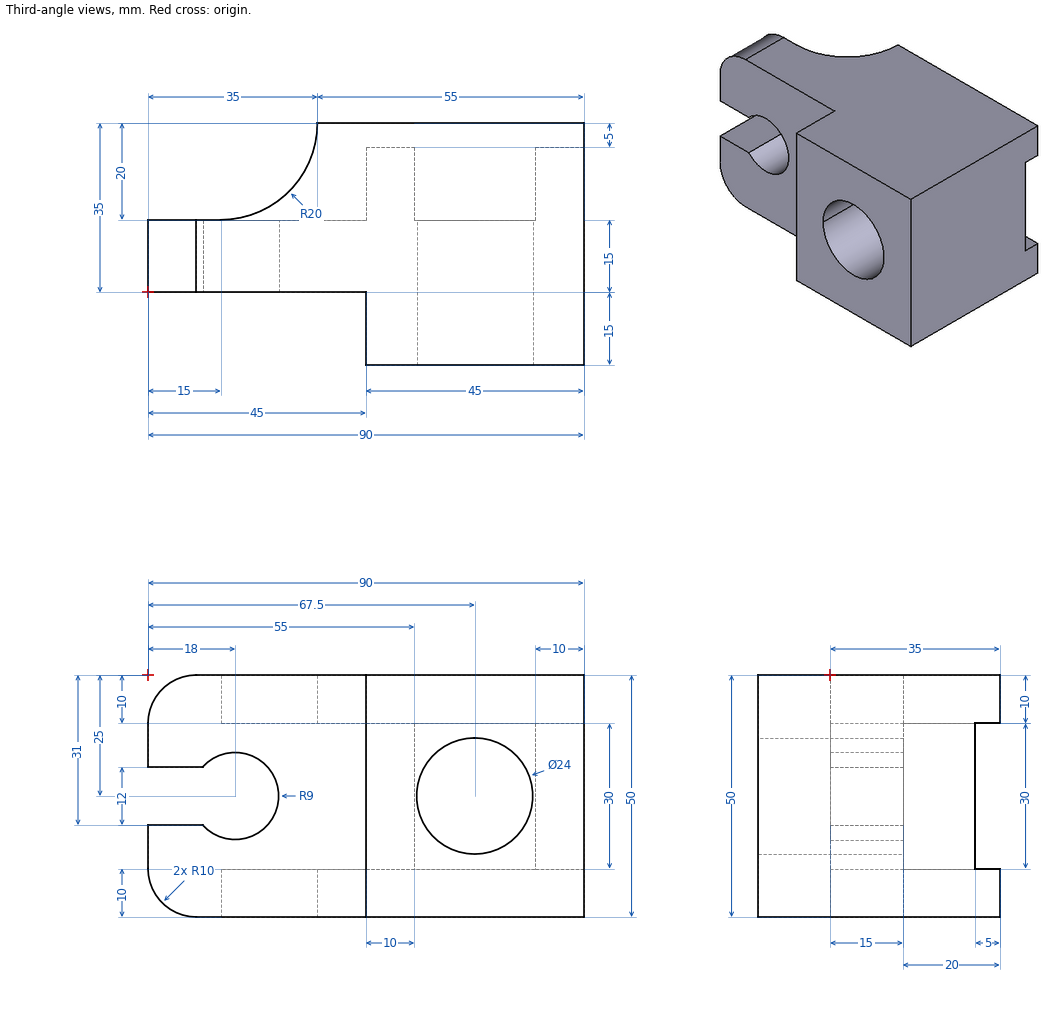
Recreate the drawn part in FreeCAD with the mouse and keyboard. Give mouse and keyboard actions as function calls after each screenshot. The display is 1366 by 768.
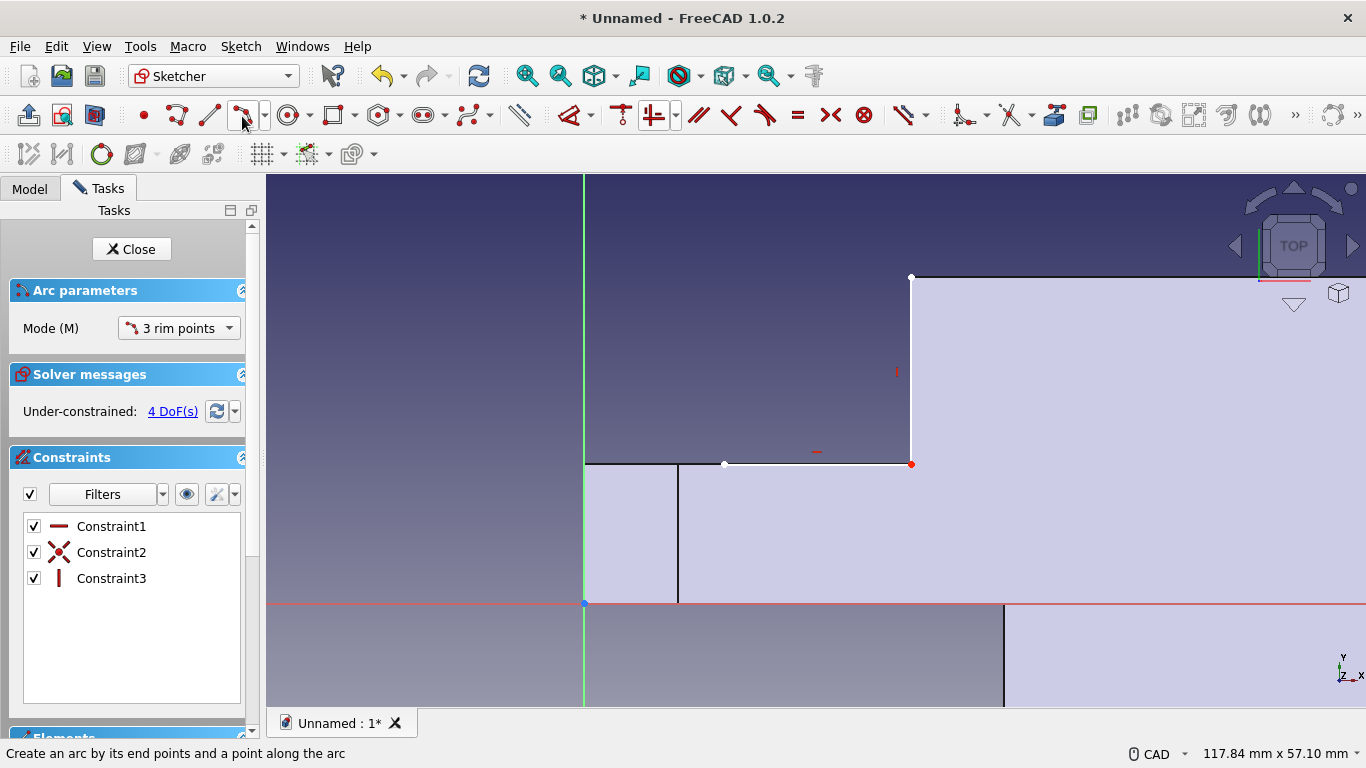
click(911, 278)
click(724, 465)
click(856, 409)
key(Escape)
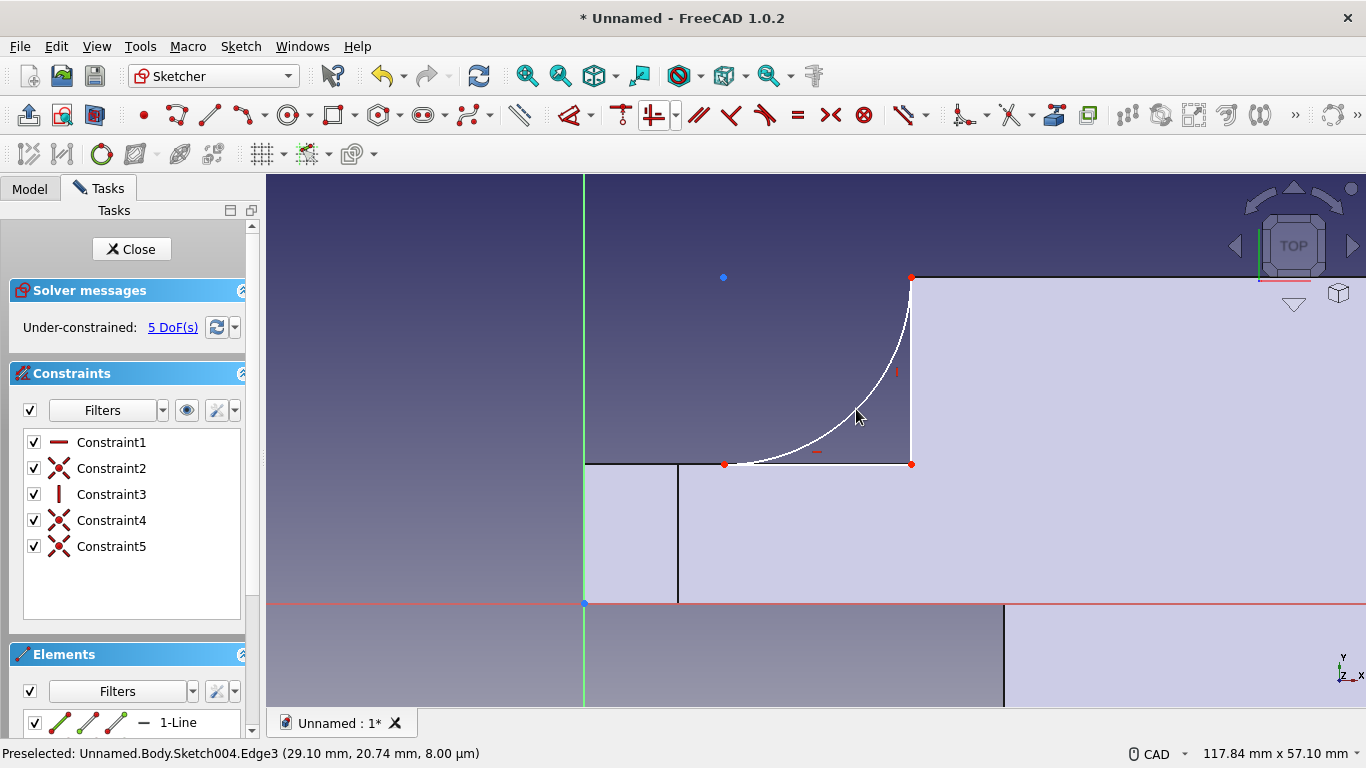
click(855, 465)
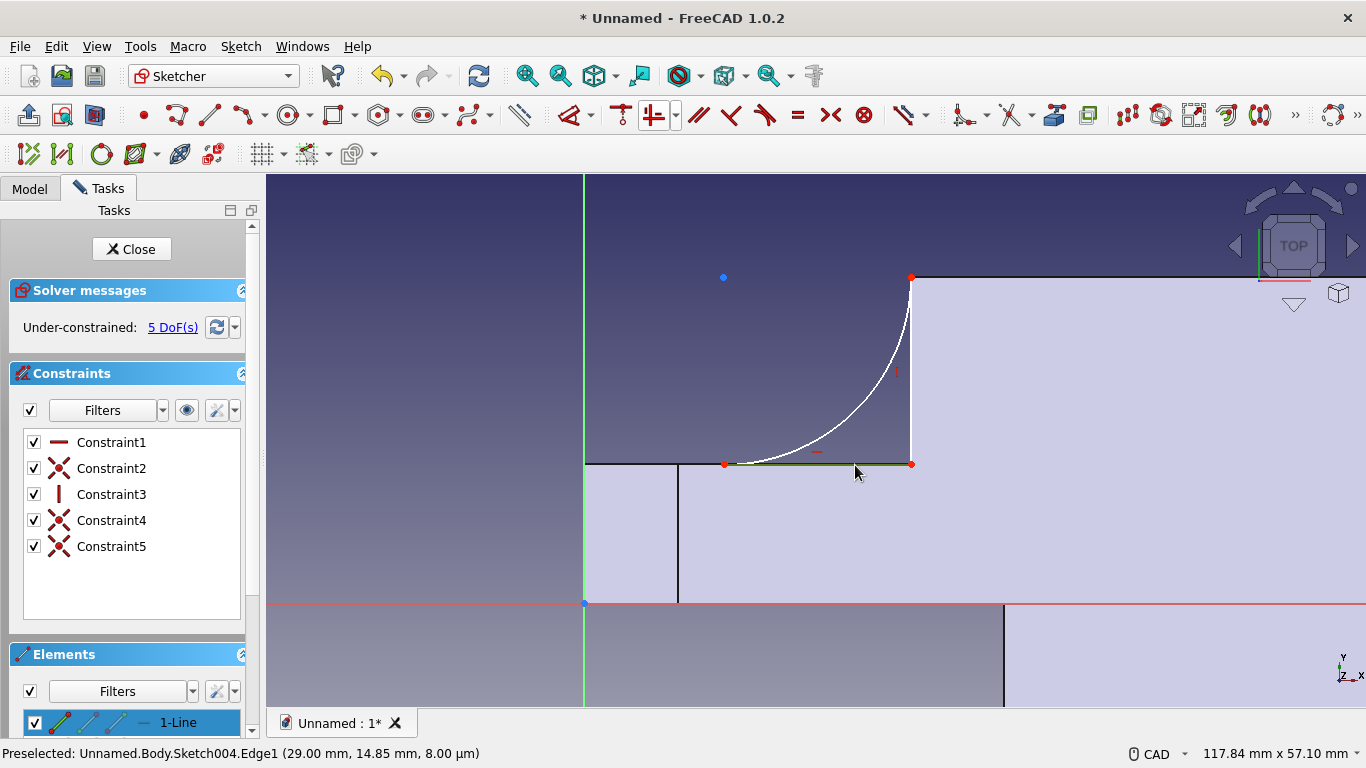
click(809, 444)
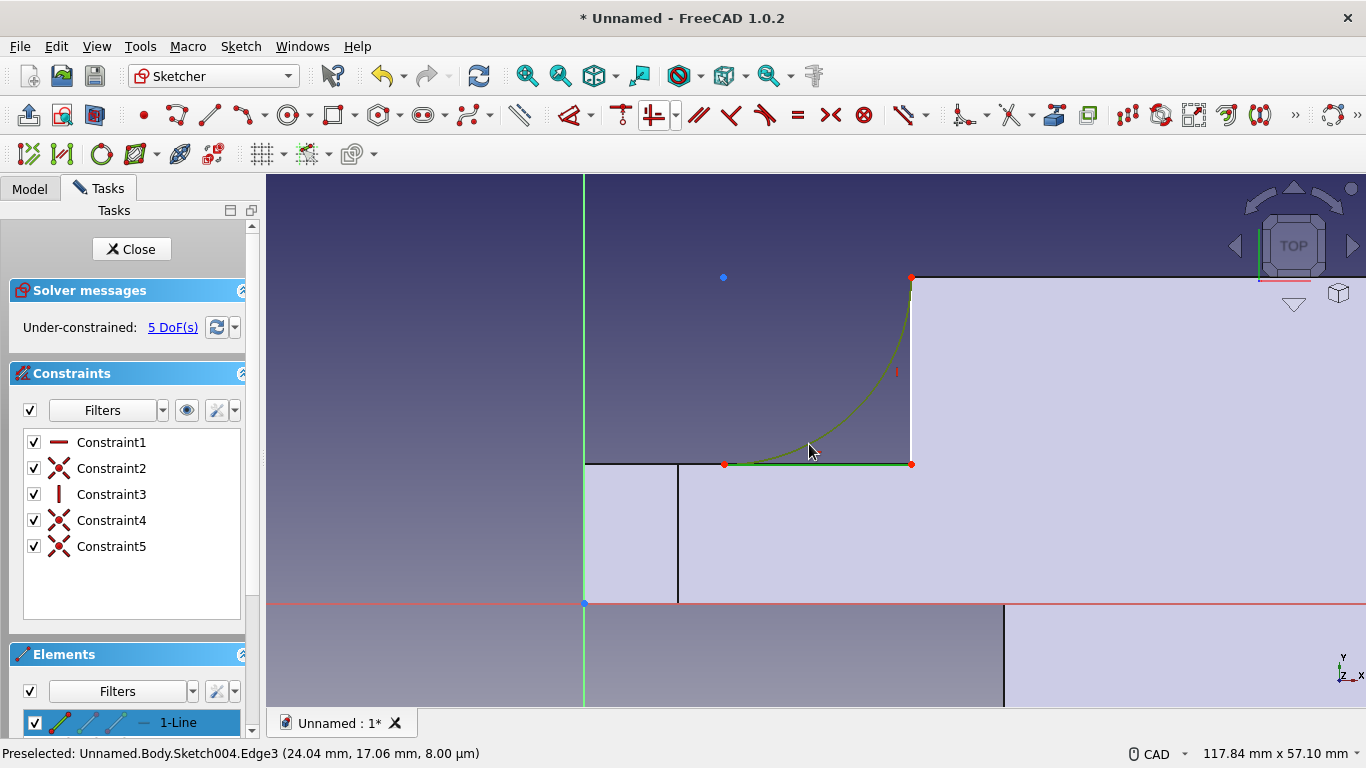
click(765, 116)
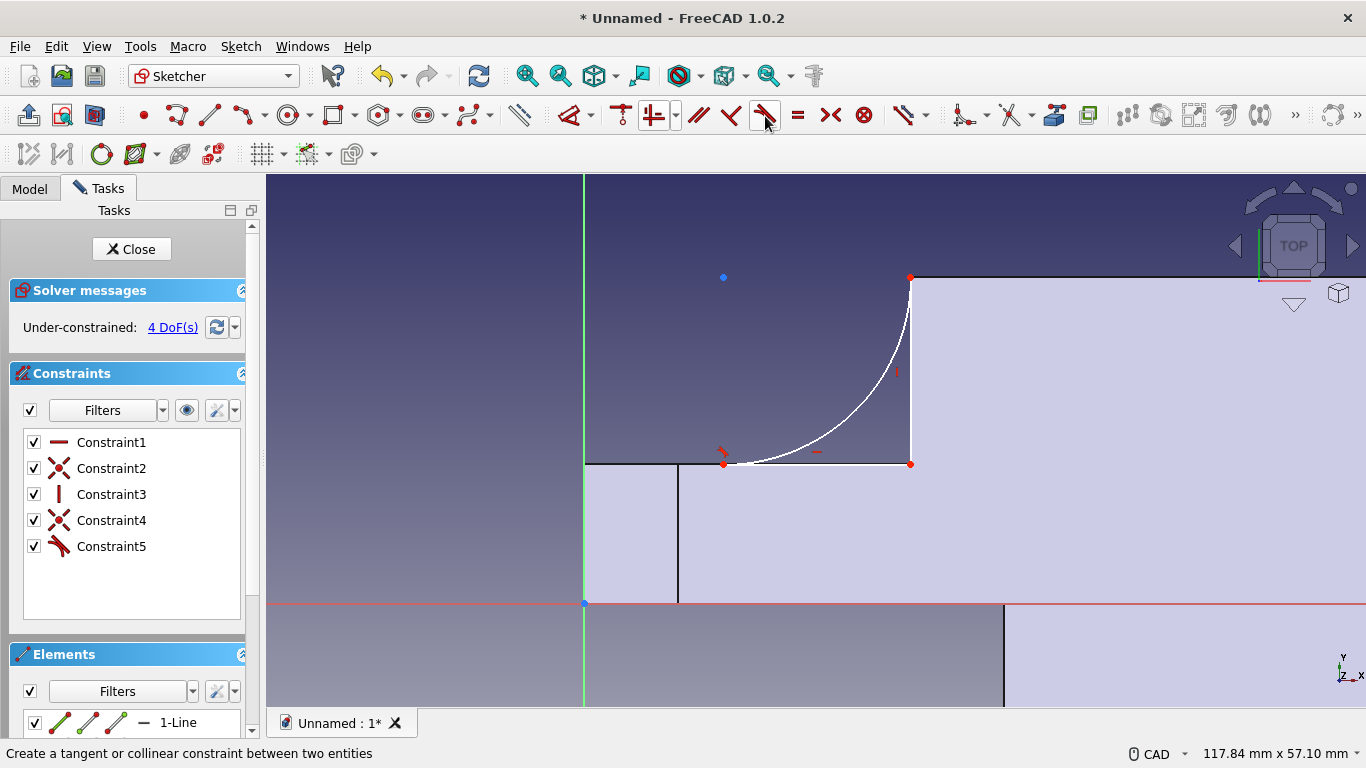
click(911, 409)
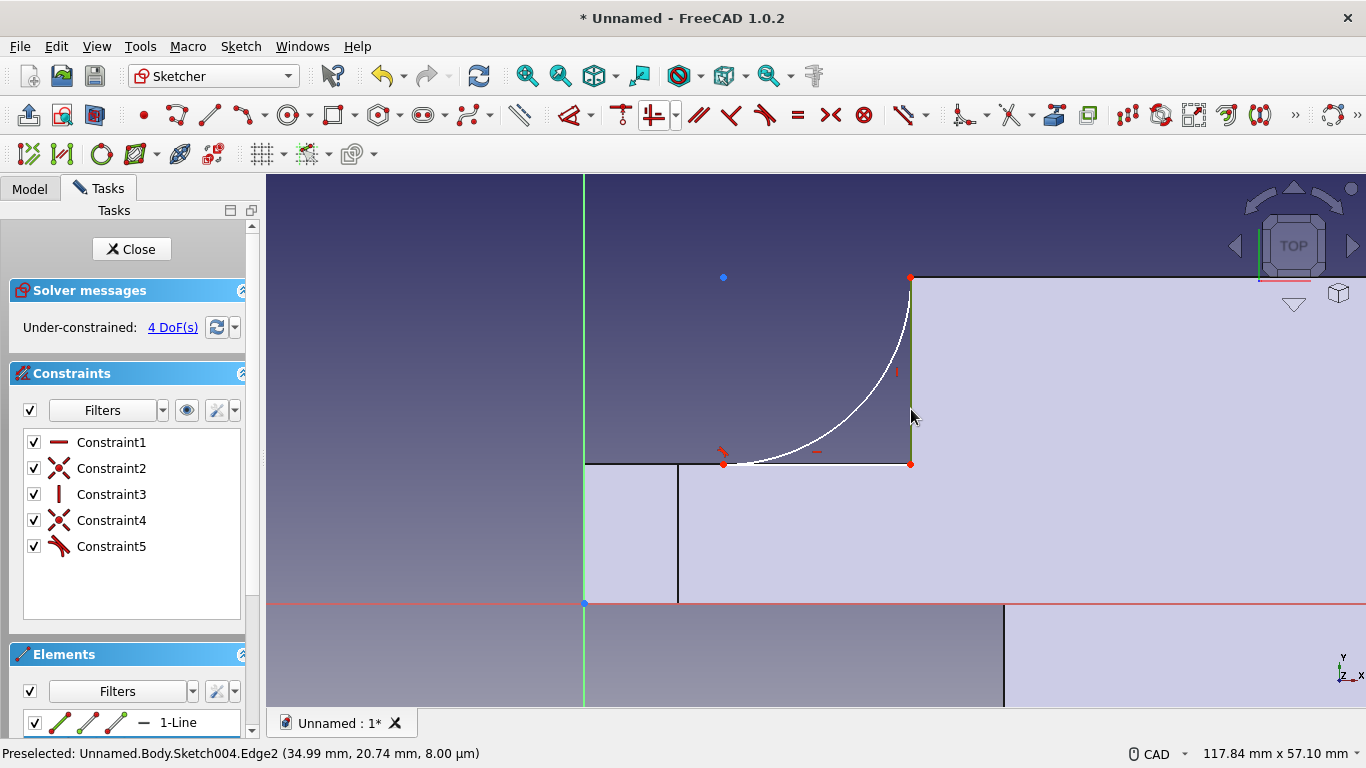
click(808, 445)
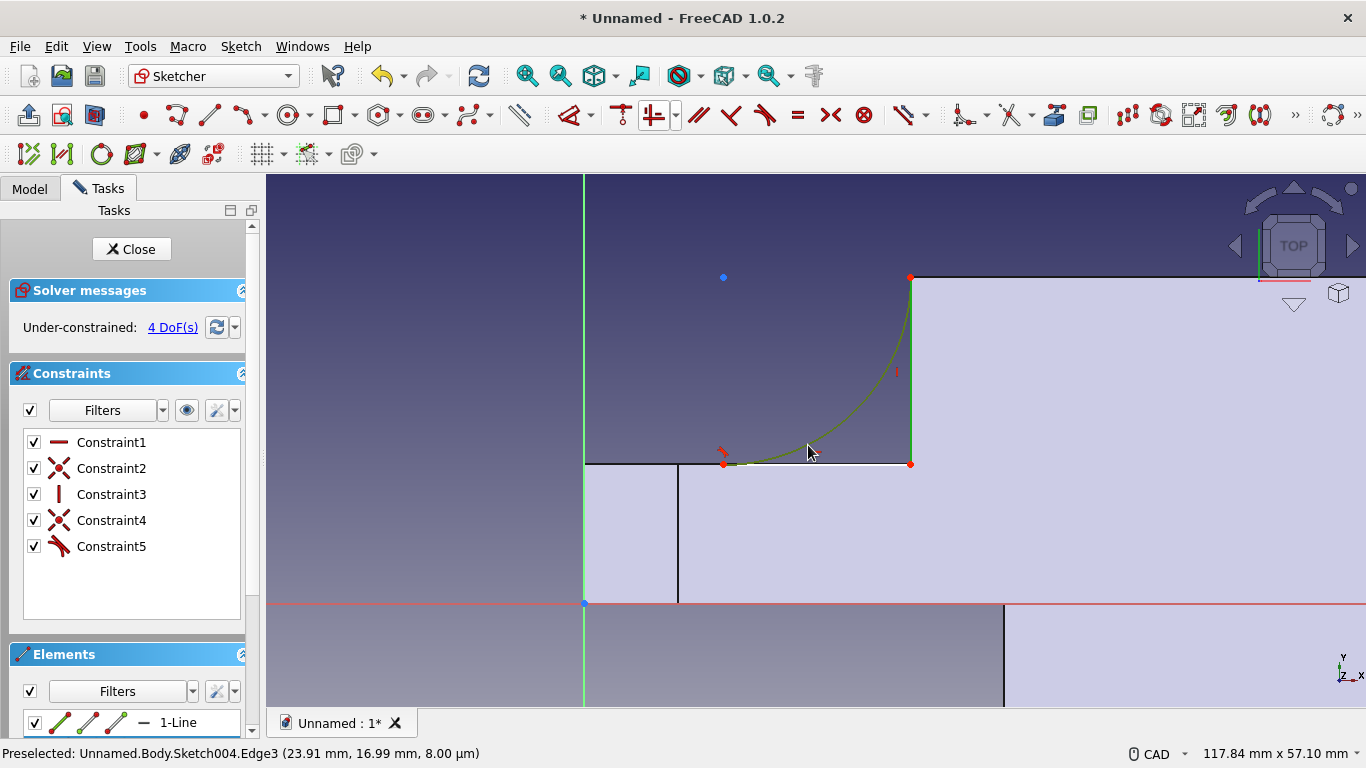
click(765, 116)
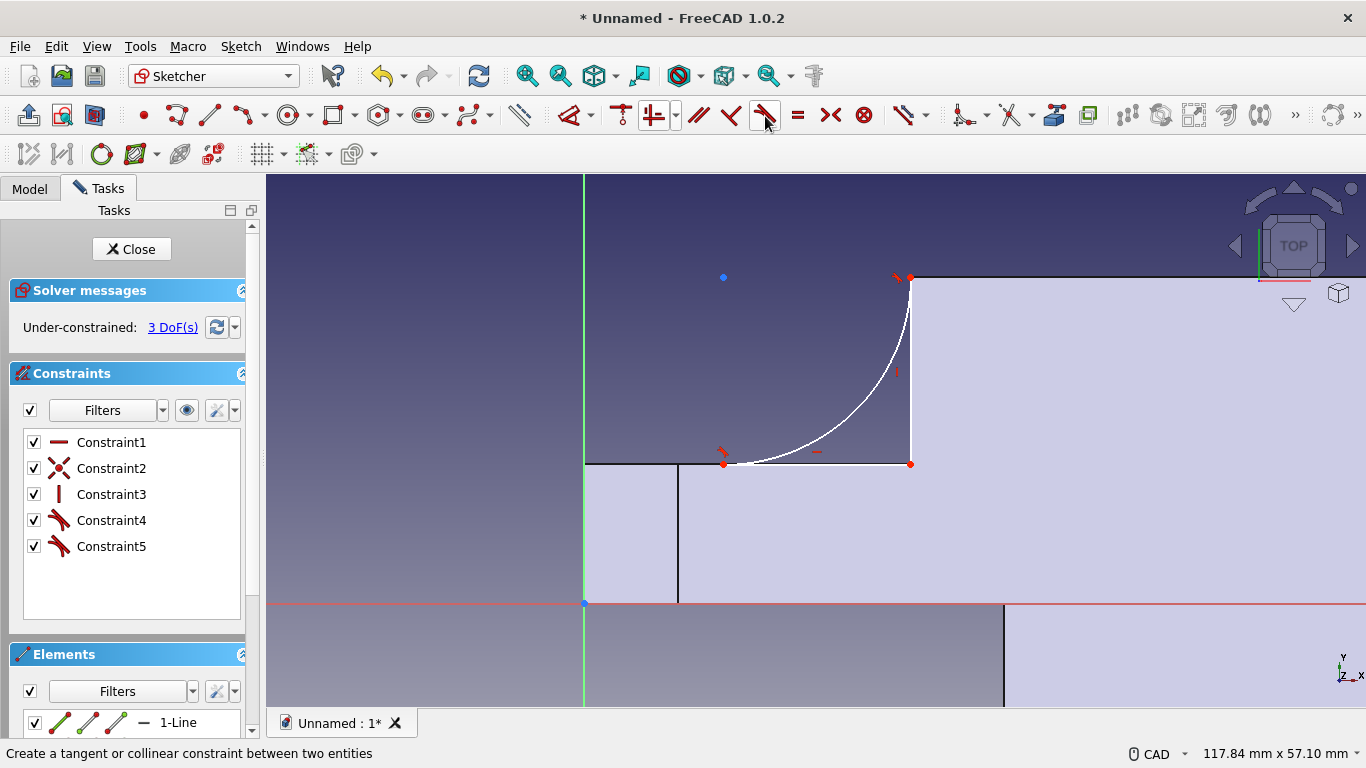
click(568, 116)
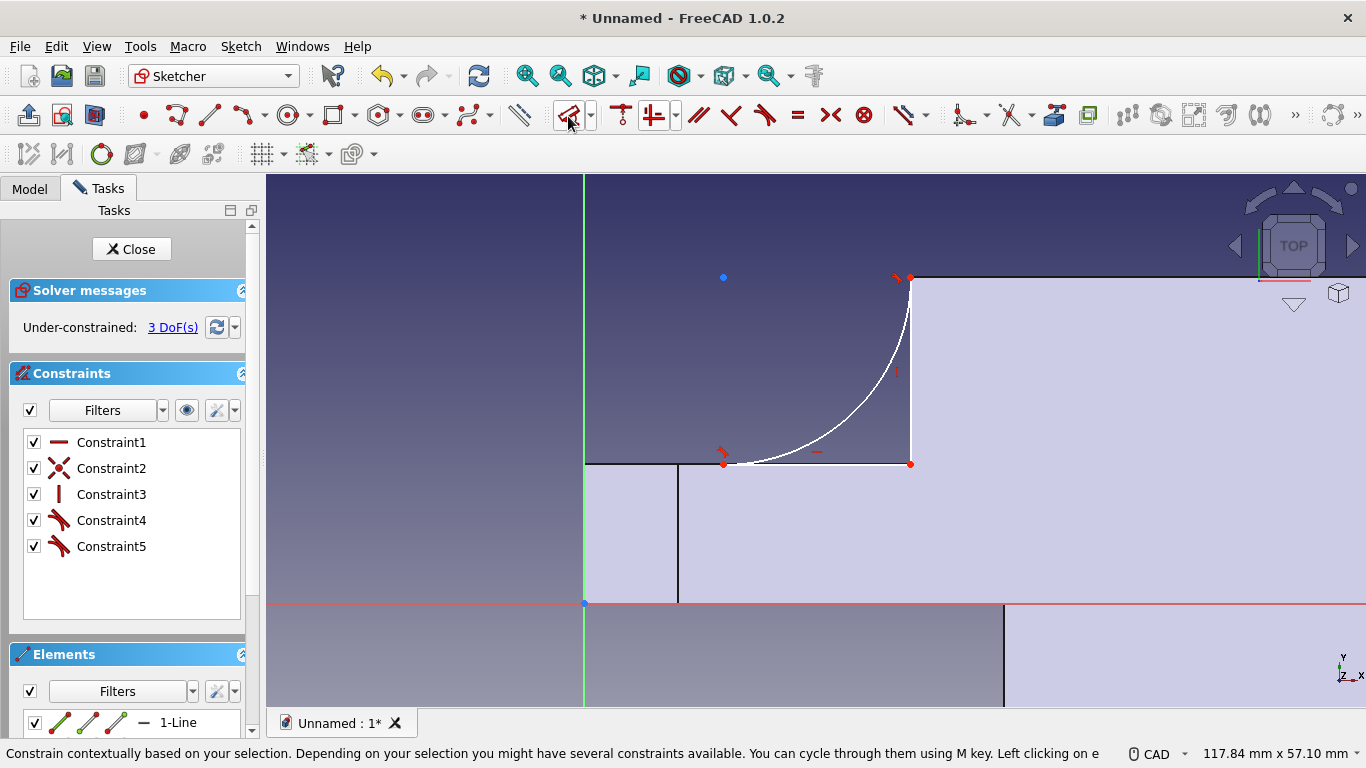
click(808, 445)
click(716, 497)